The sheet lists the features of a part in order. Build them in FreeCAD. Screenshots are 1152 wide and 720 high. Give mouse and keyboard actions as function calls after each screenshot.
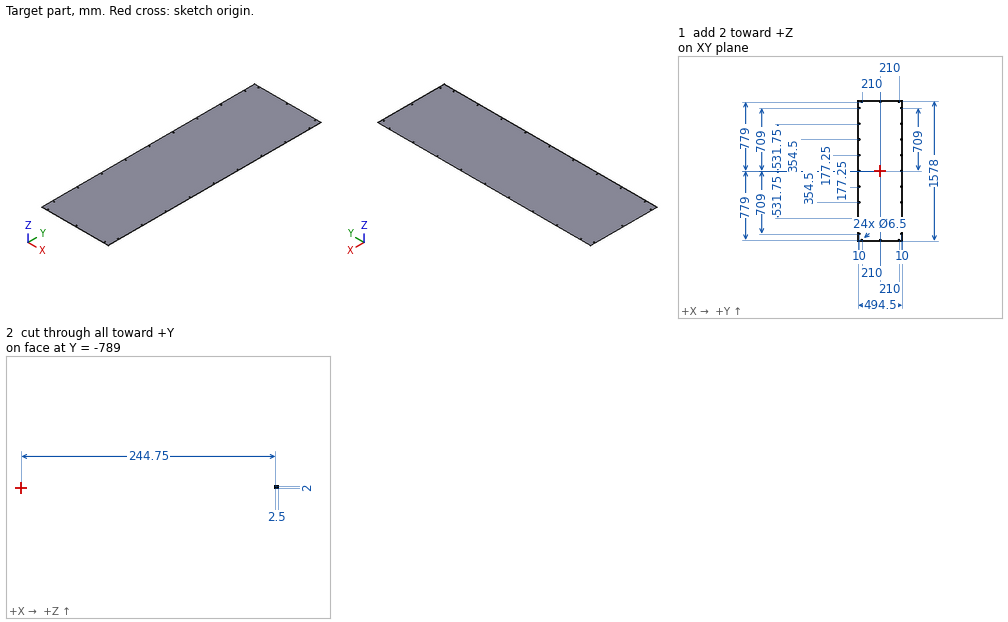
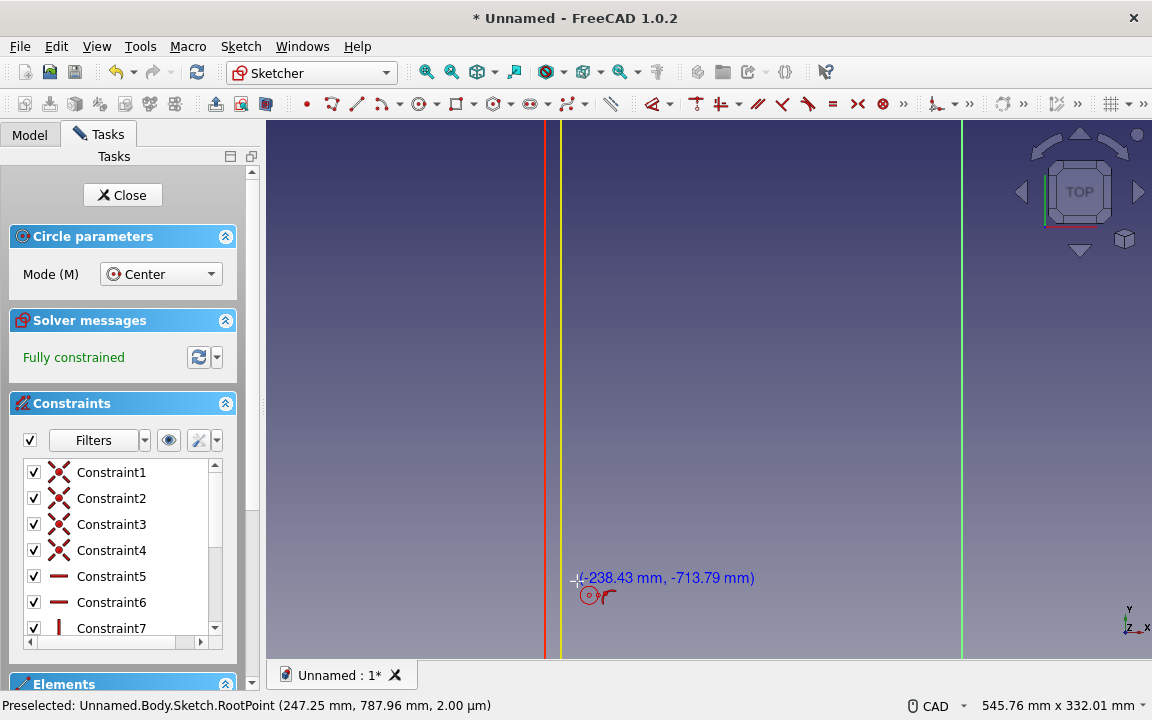
click(577, 575)
move(581, 571)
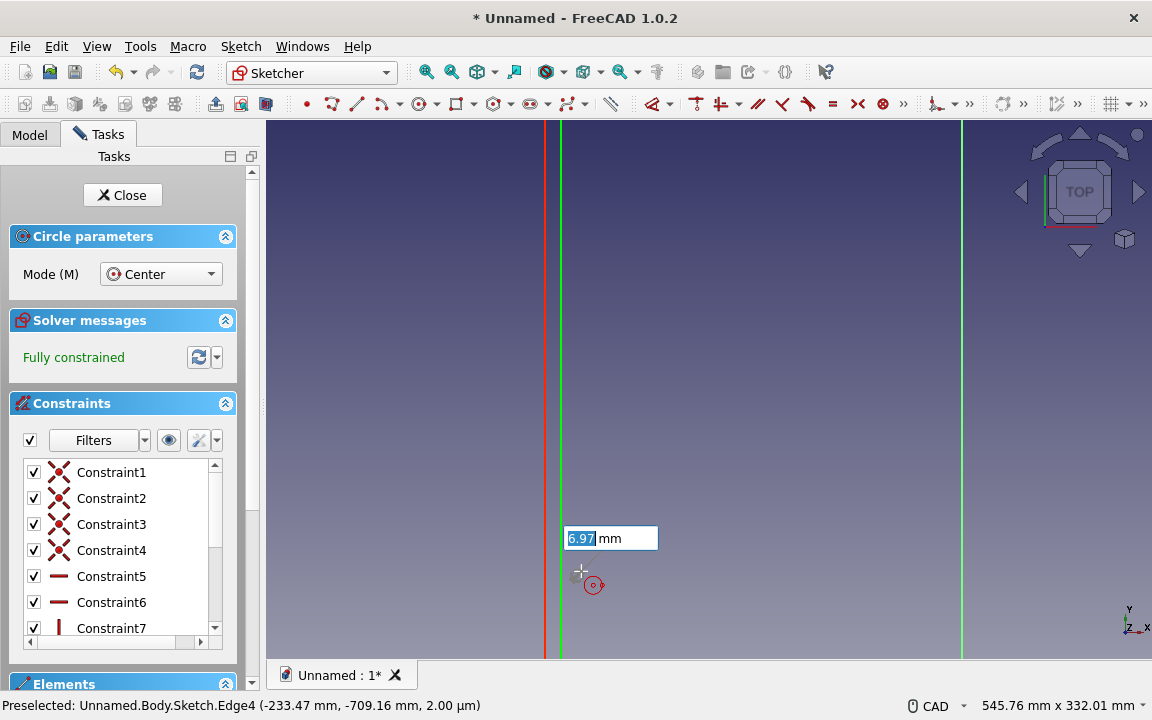
text(6.5)
key(Return)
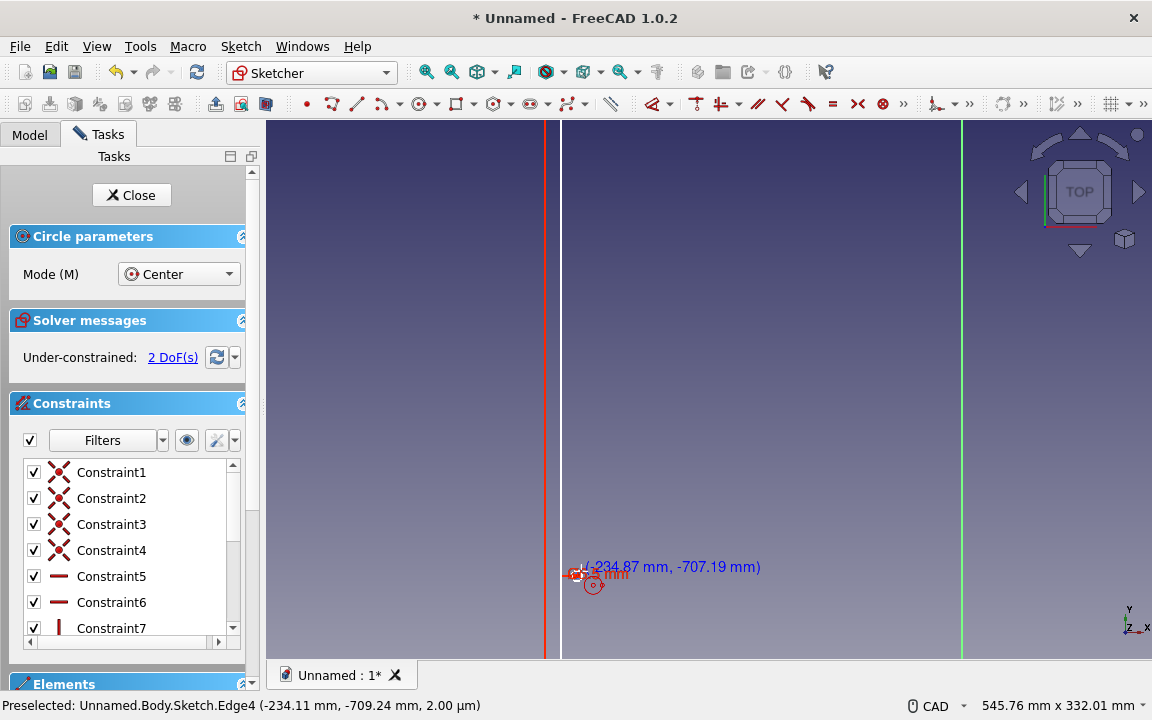
scroll(590, 541, down, 10)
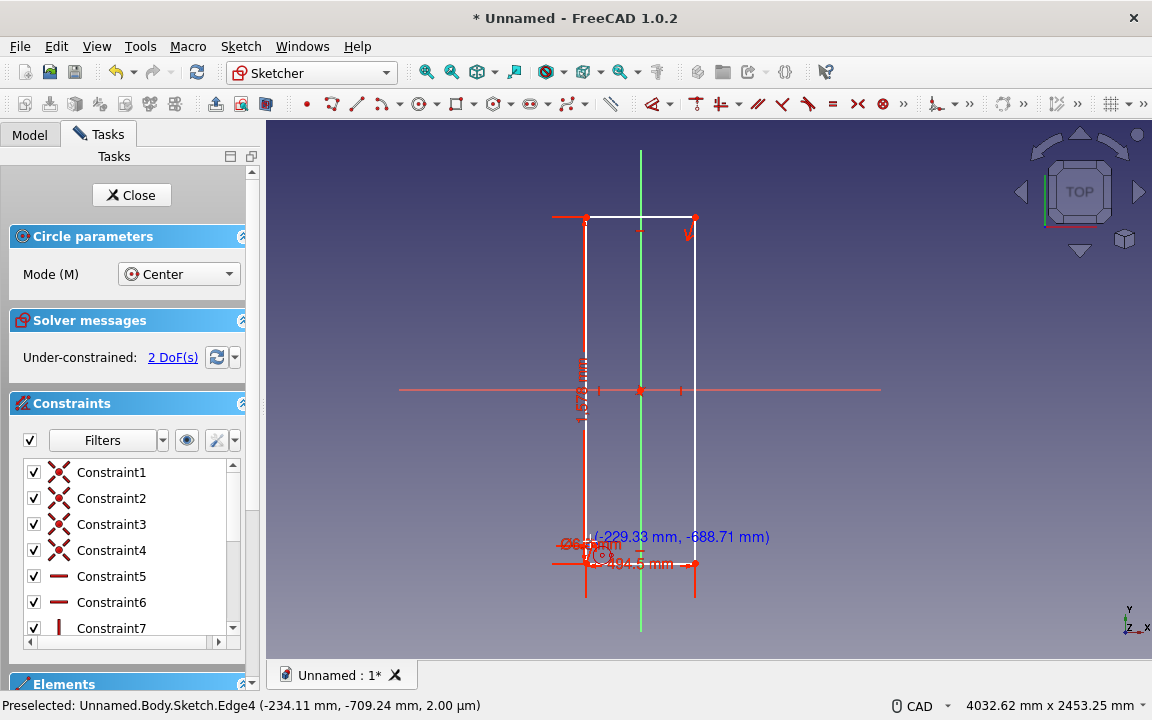
scroll(595, 562, up, 18)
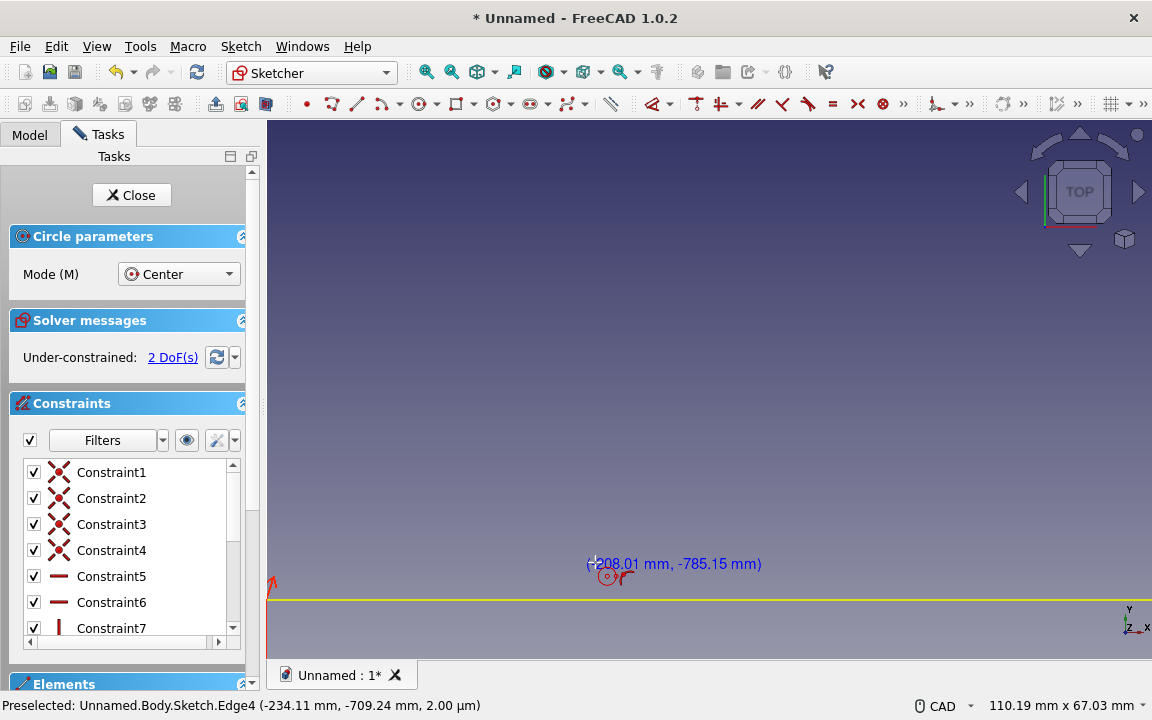
scroll(585, 601, down, 17)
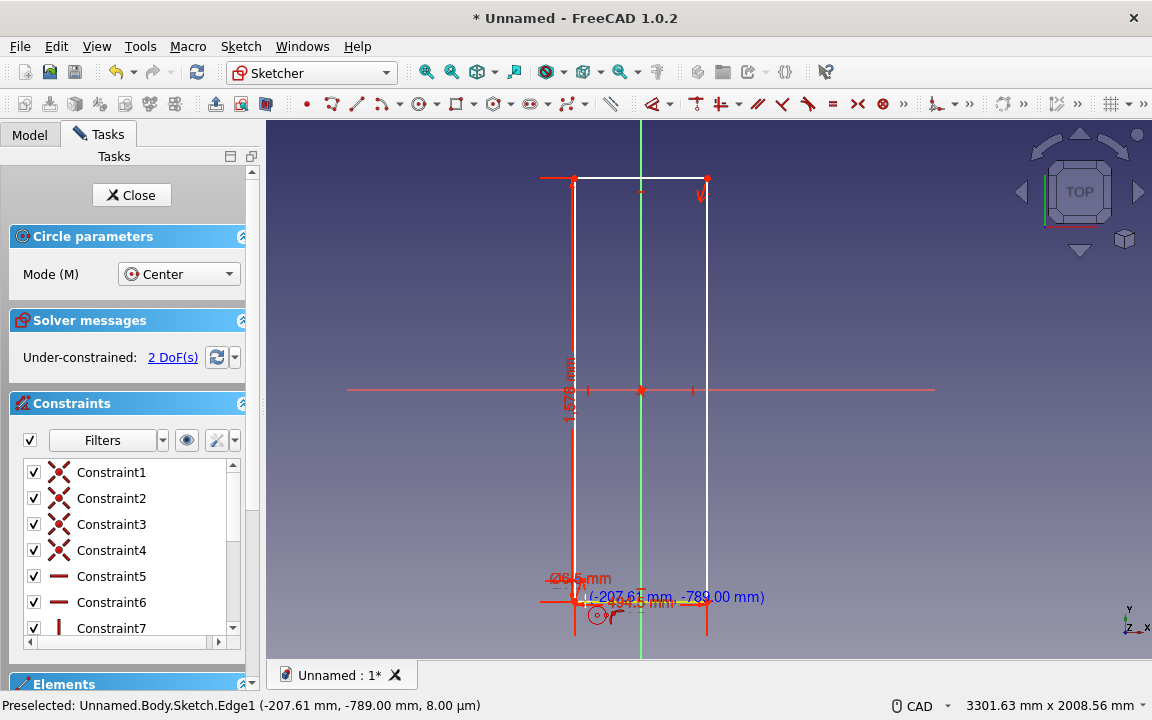
scroll(585, 599, up, 9)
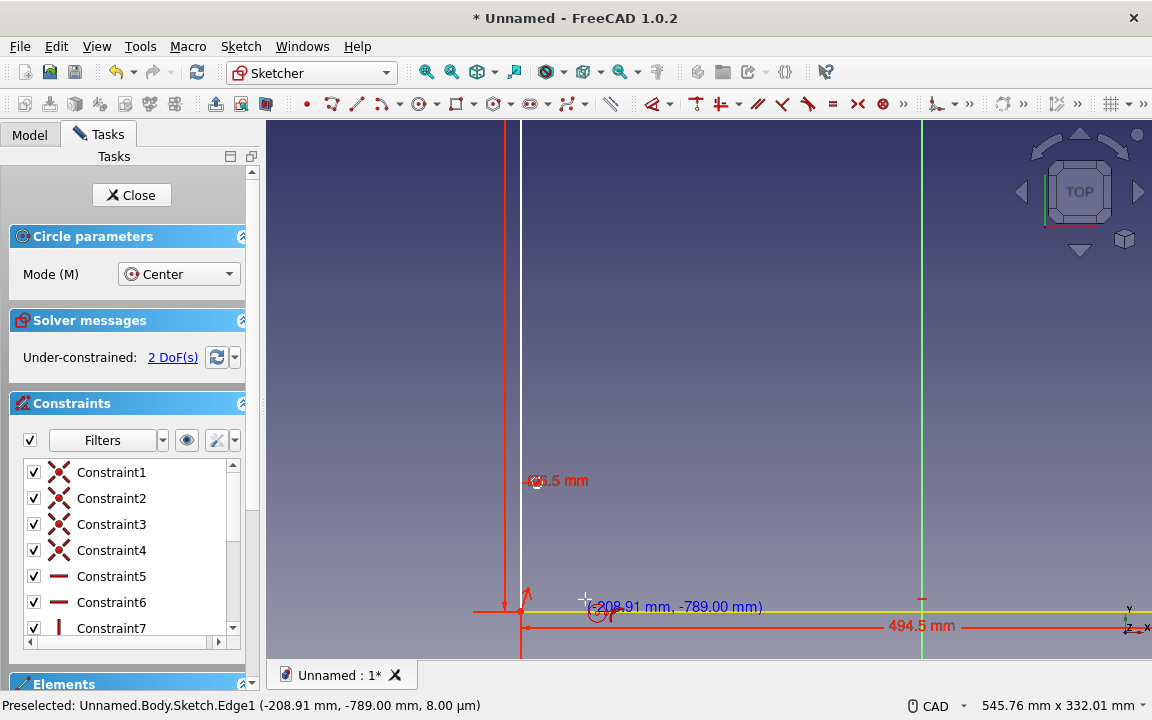
click(581, 595)
move(585, 592)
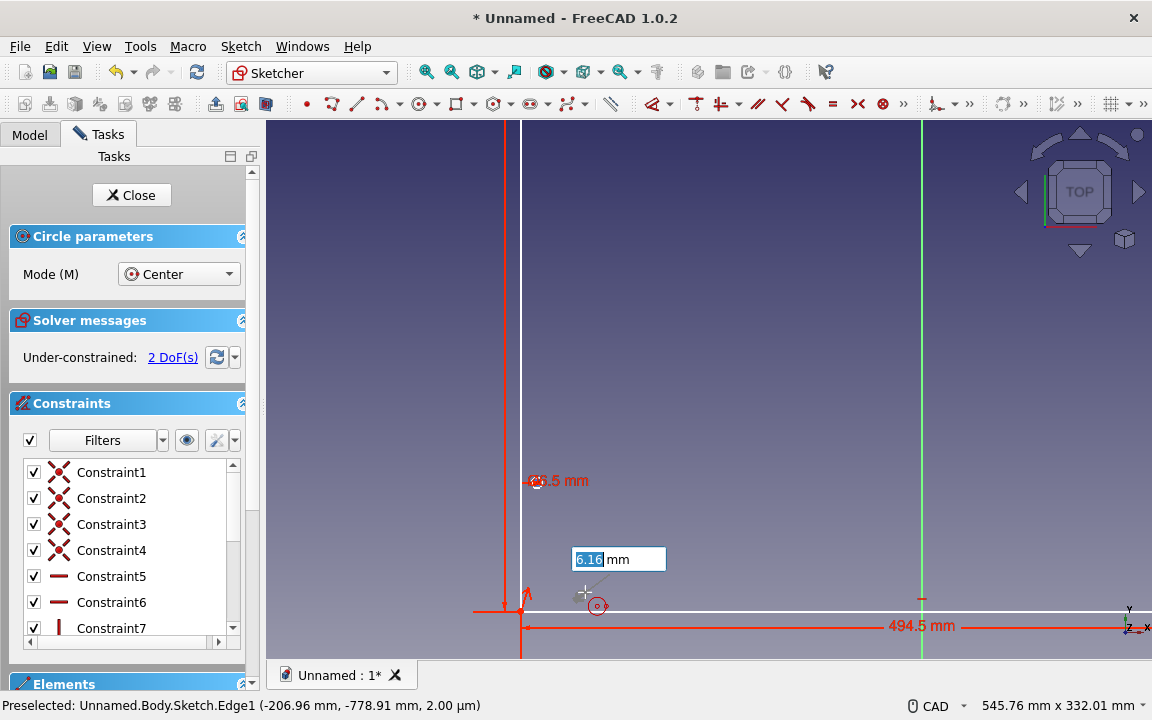
text(6.5)
key(Return)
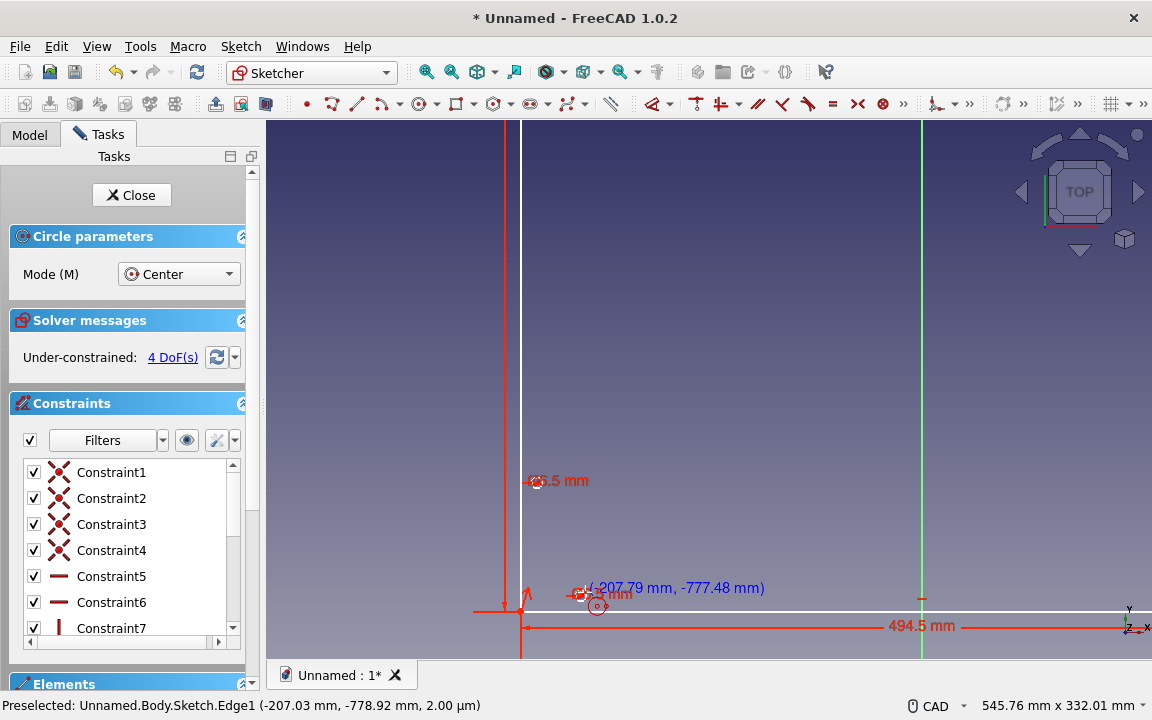
scroll(537, 194, up, 8)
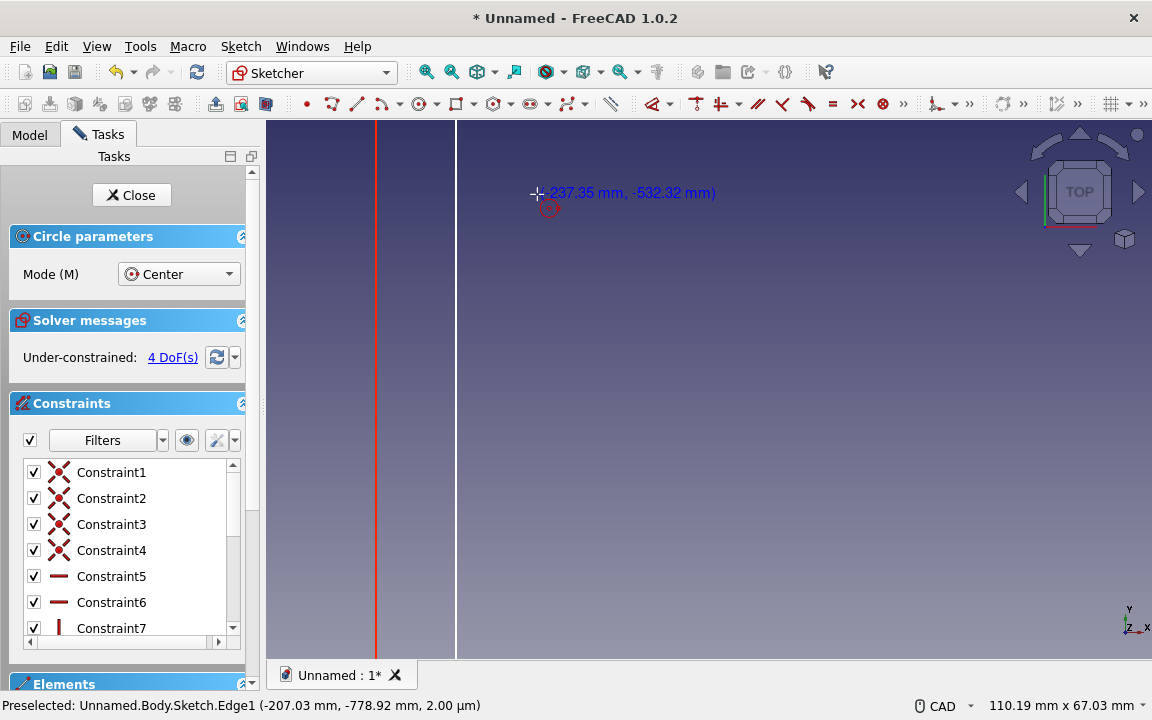
scroll(578, 544, down, 17)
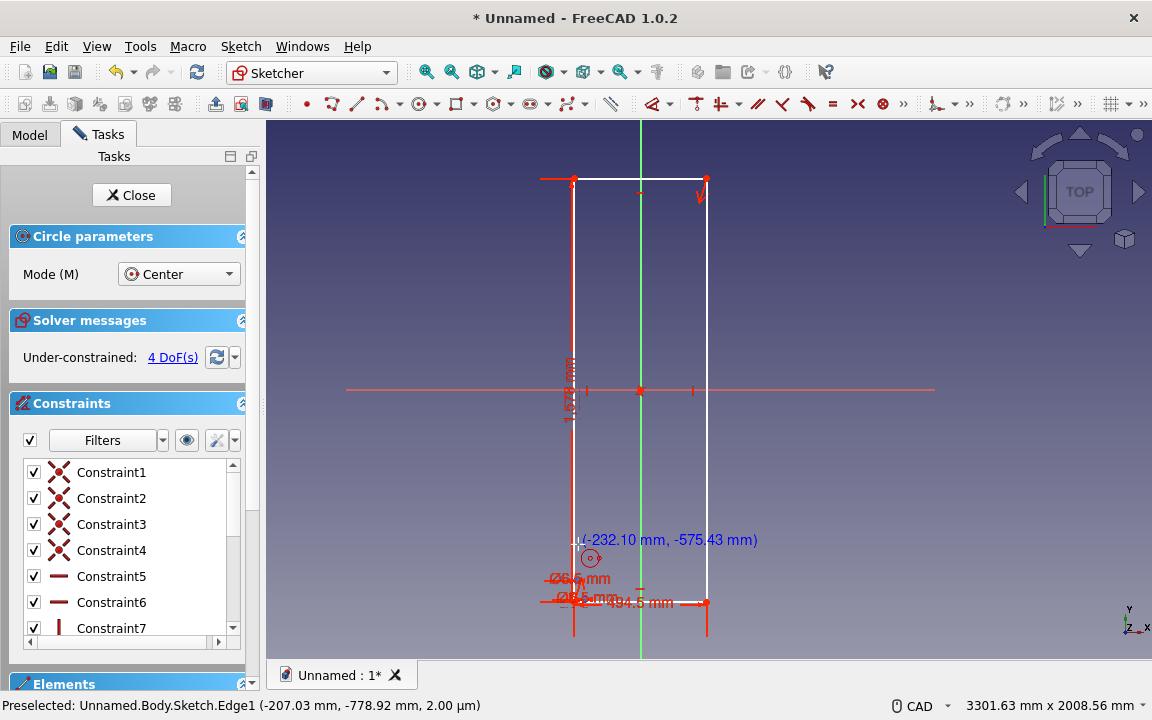
scroll(577, 533, up, 9)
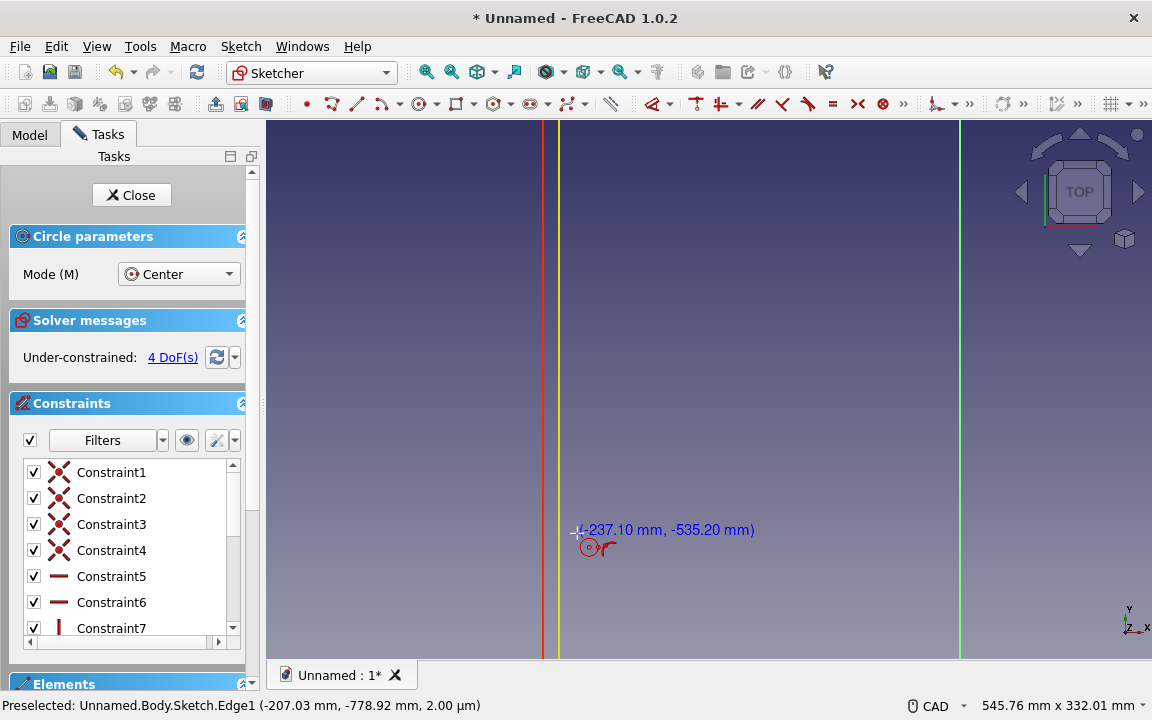
click(575, 530)
move(579, 526)